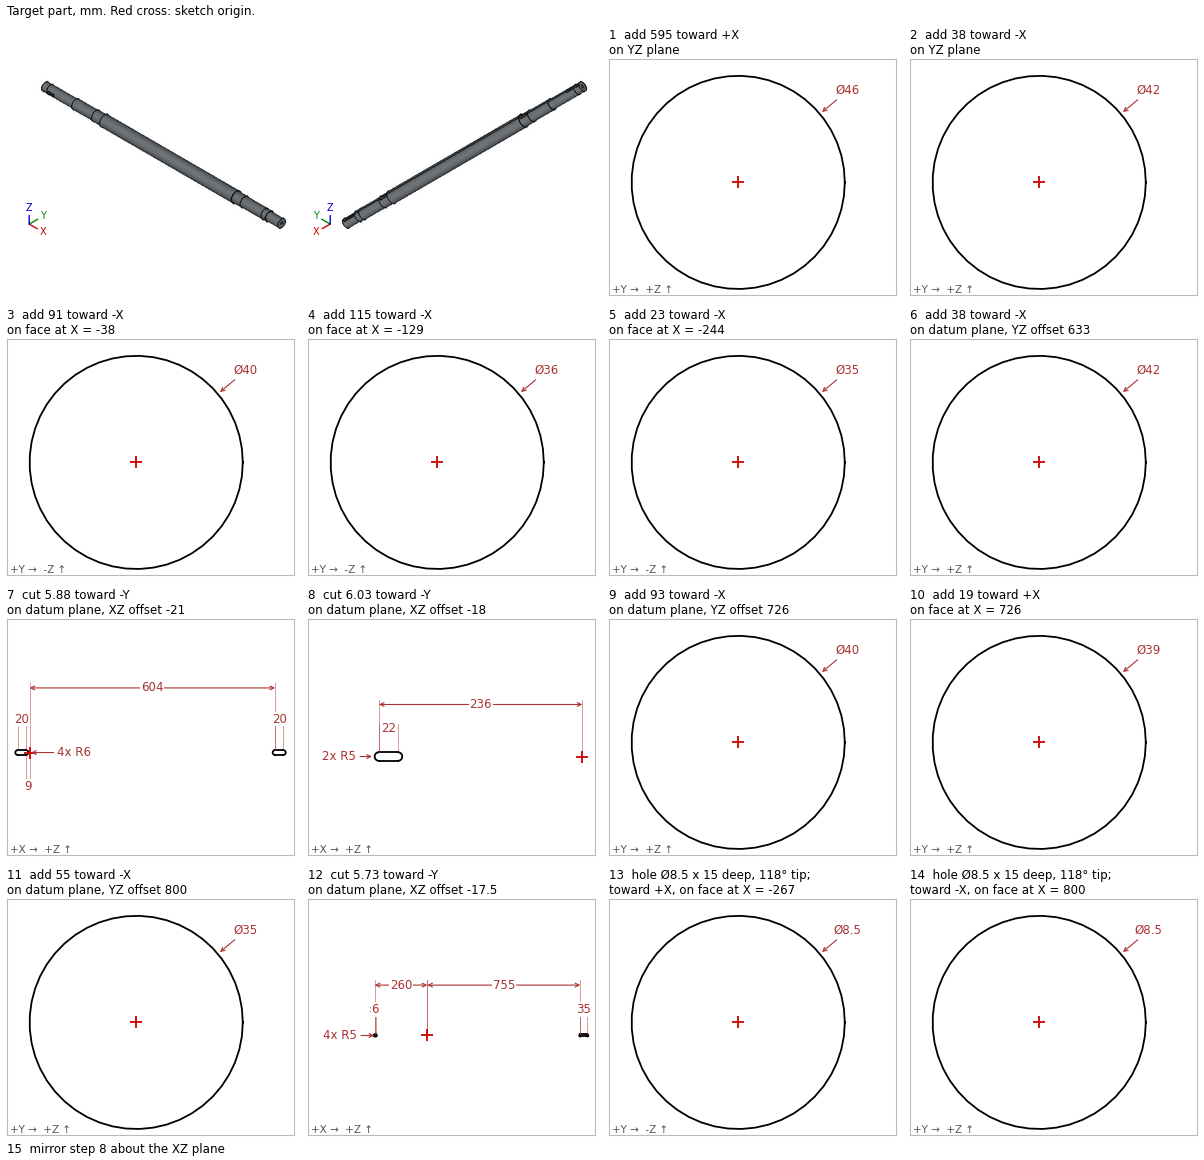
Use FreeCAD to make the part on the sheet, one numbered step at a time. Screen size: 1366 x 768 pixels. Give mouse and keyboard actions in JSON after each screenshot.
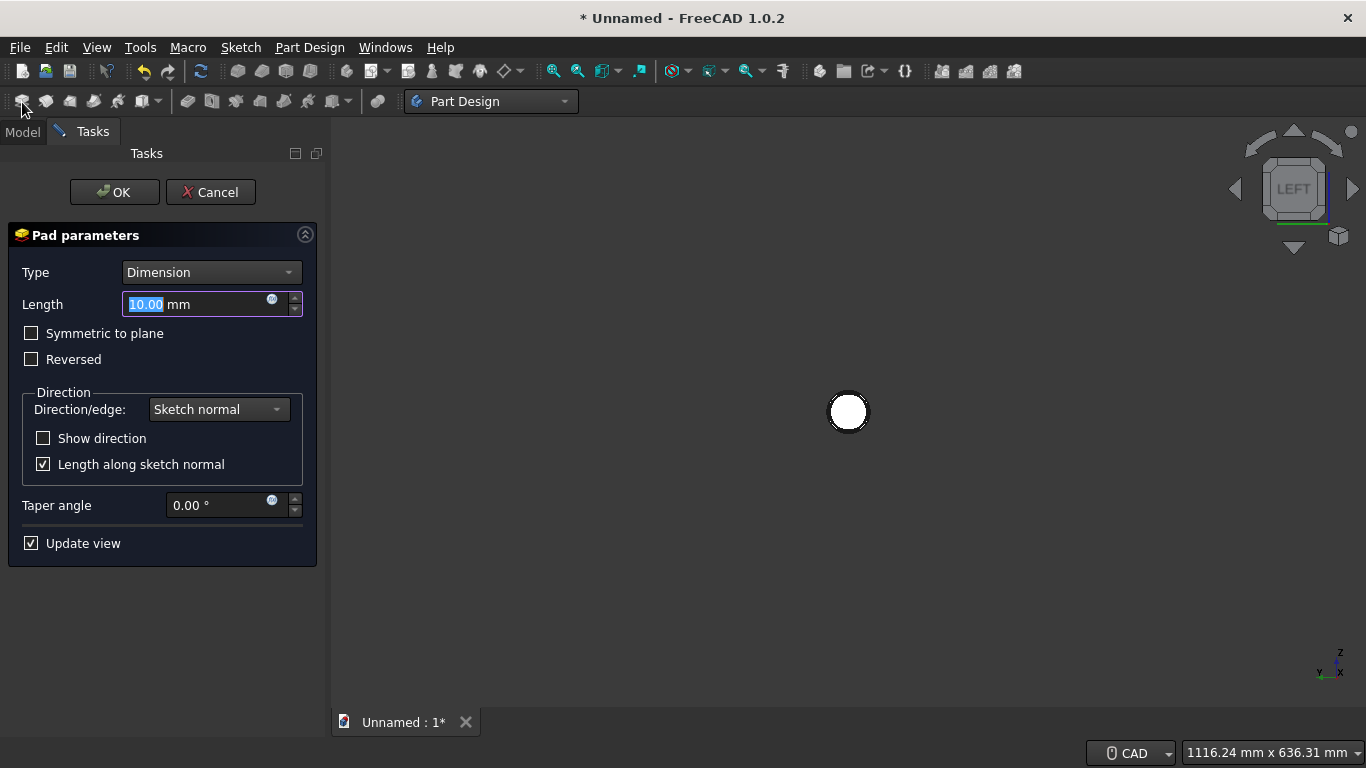
{"action": "type", "text": "91"}
{"action": "key", "text": "Tab"}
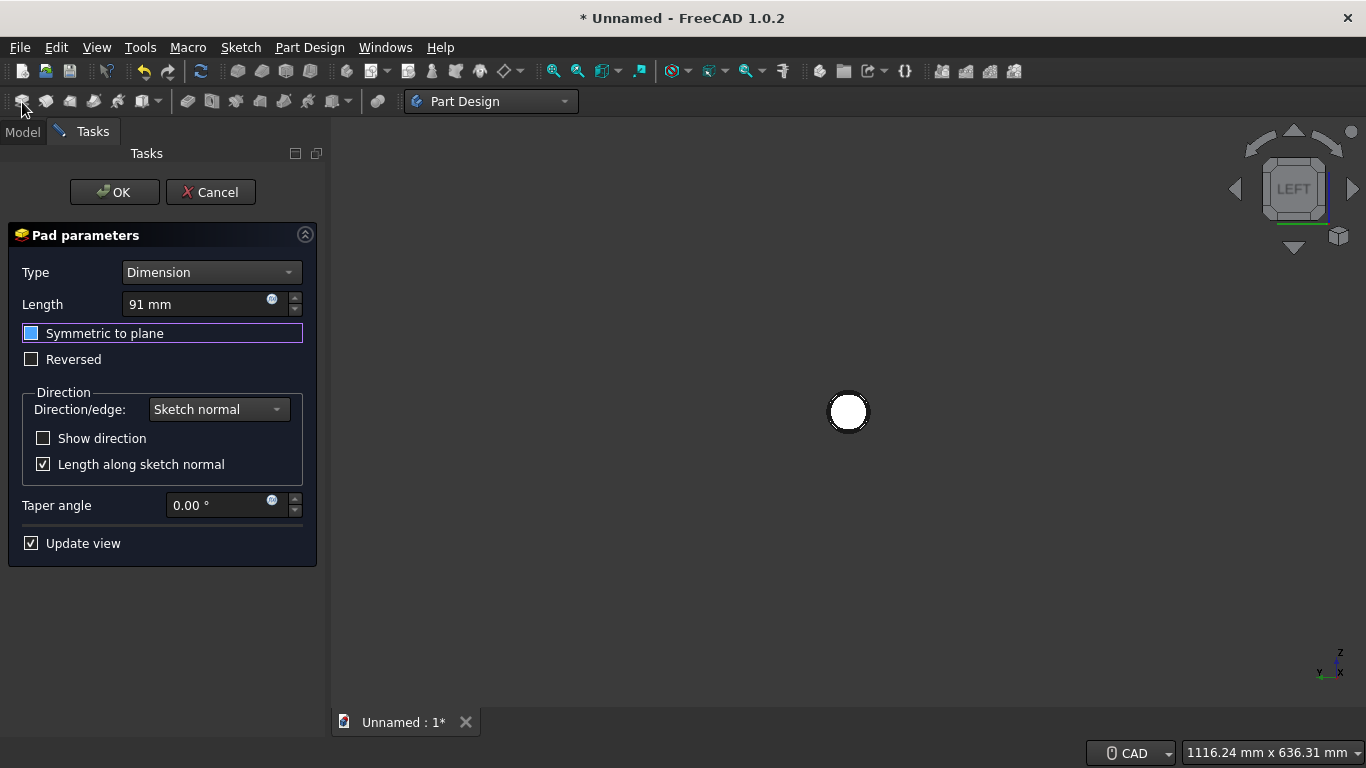
{"action": "left_click", "coordinate": [115, 192]}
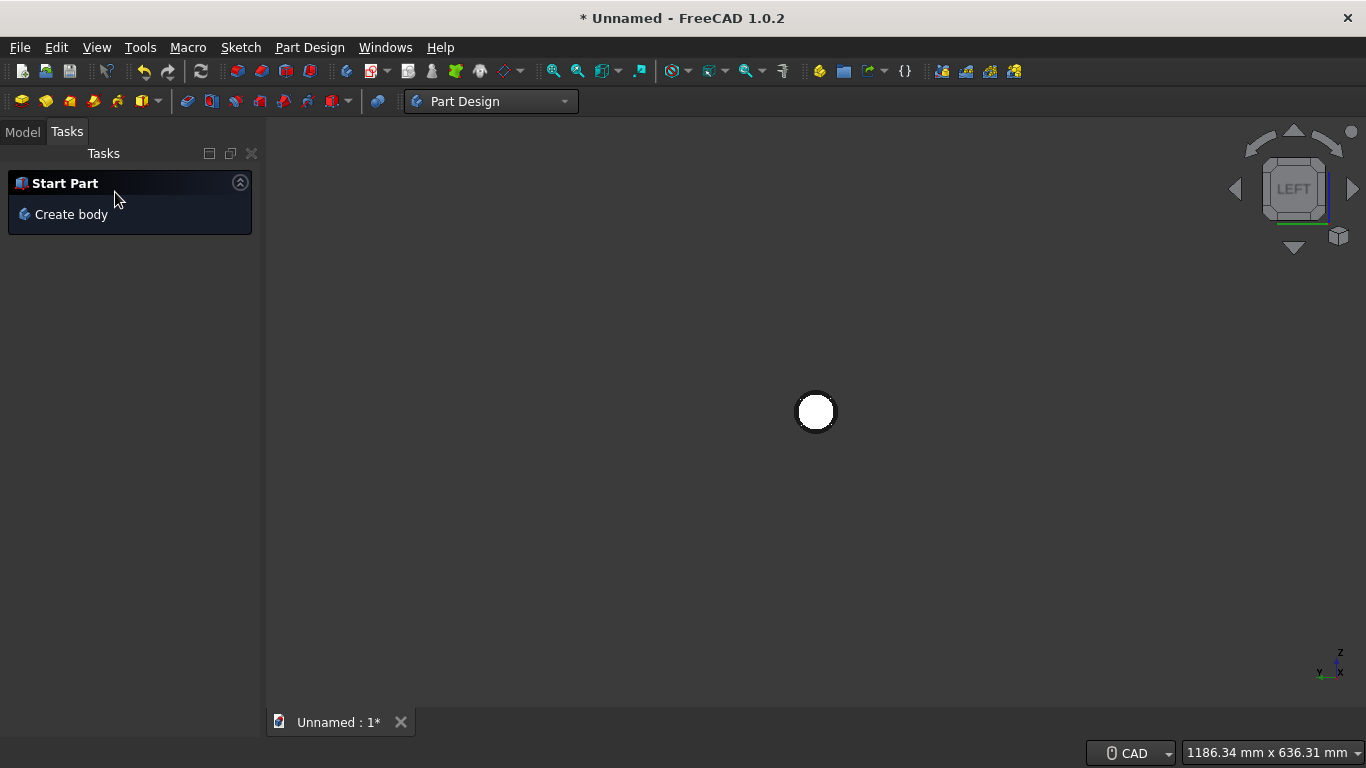
{"action": "key", "text": "v f"}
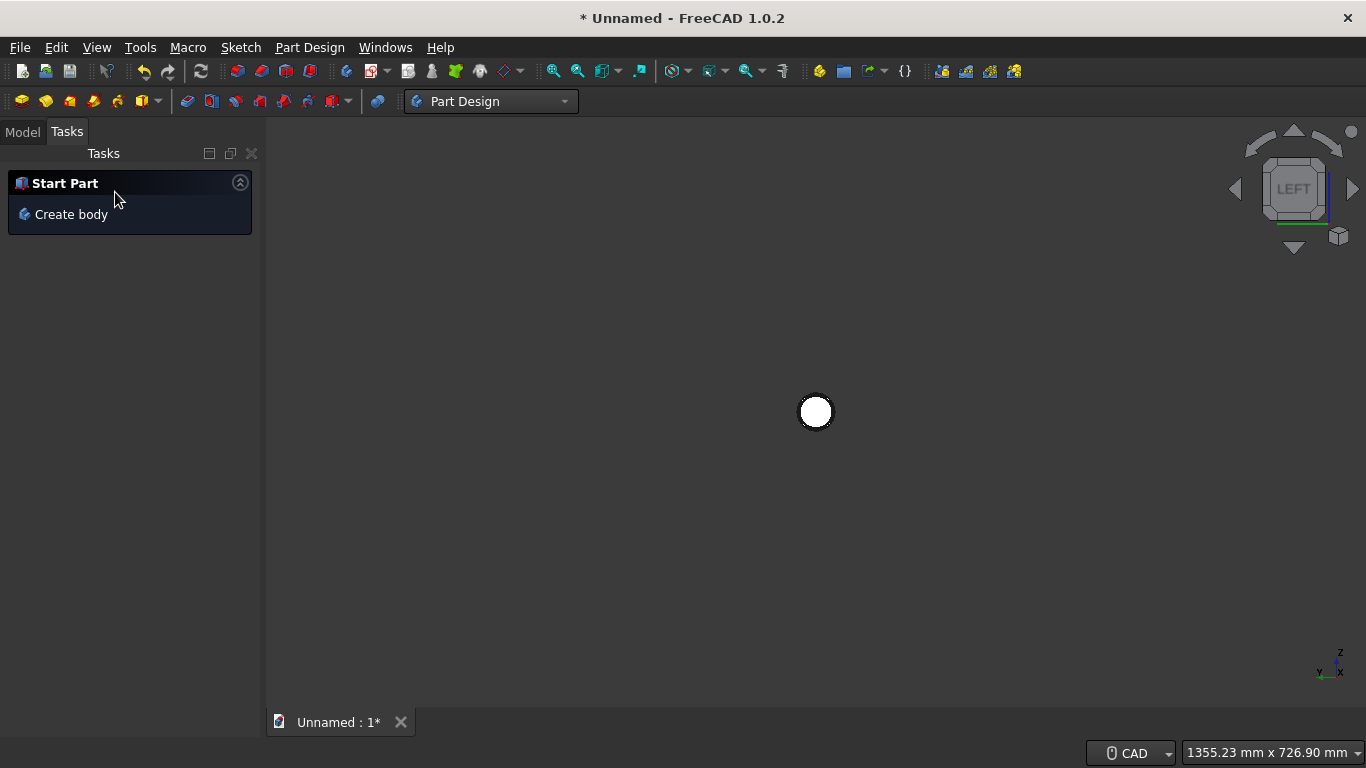
{"action": "left_click", "coordinate": [816, 411]}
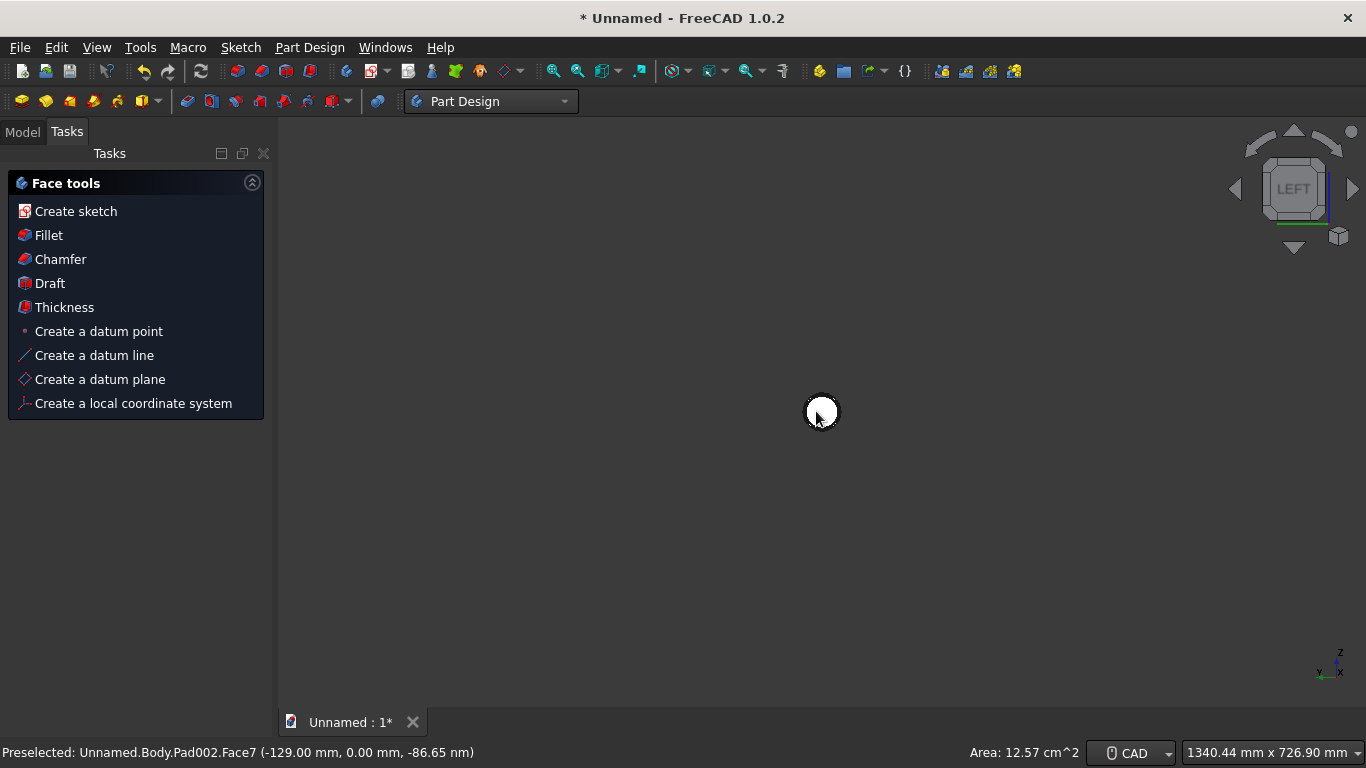
{"action": "left_click", "coordinate": [372, 72]}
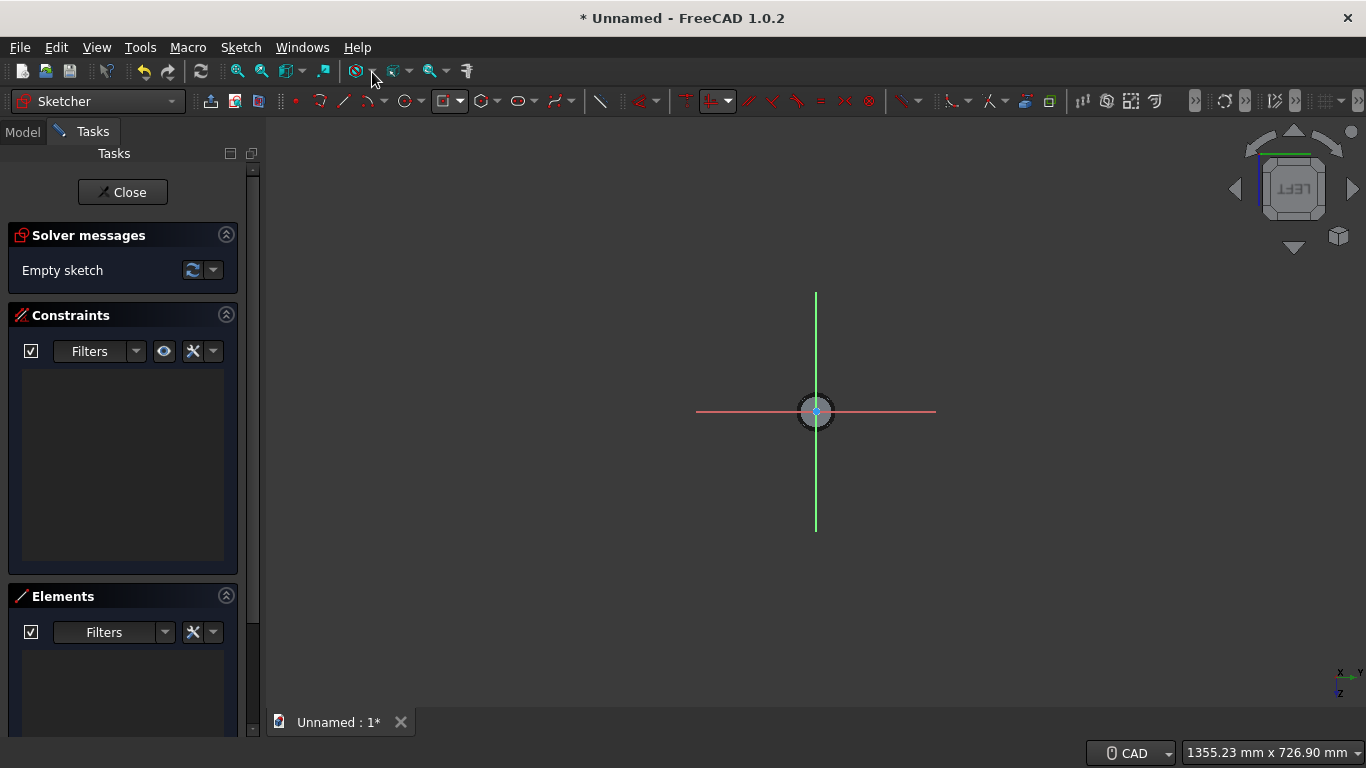
{"action": "scroll", "coordinate": [821, 412], "scroll_direction": "up", "scroll_amount": 13}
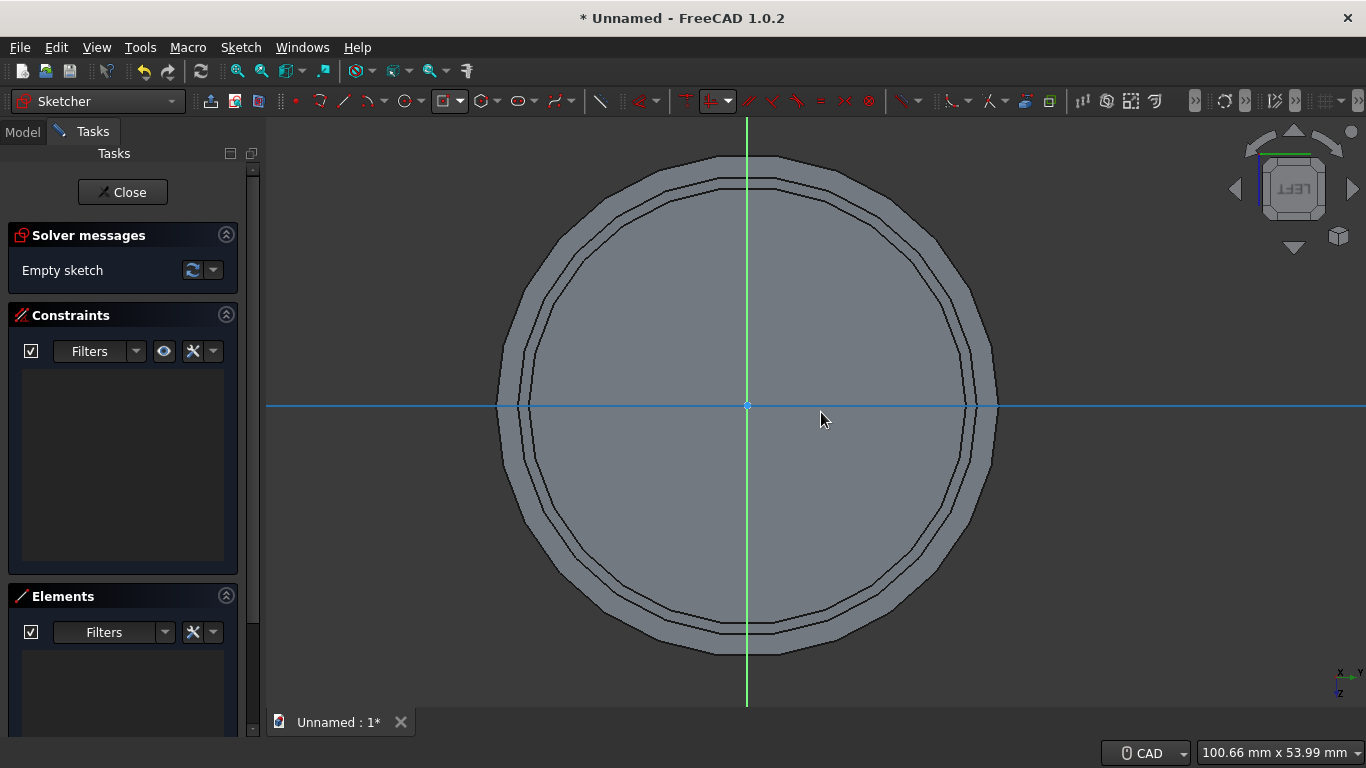
{"action": "key", "text": "g c"}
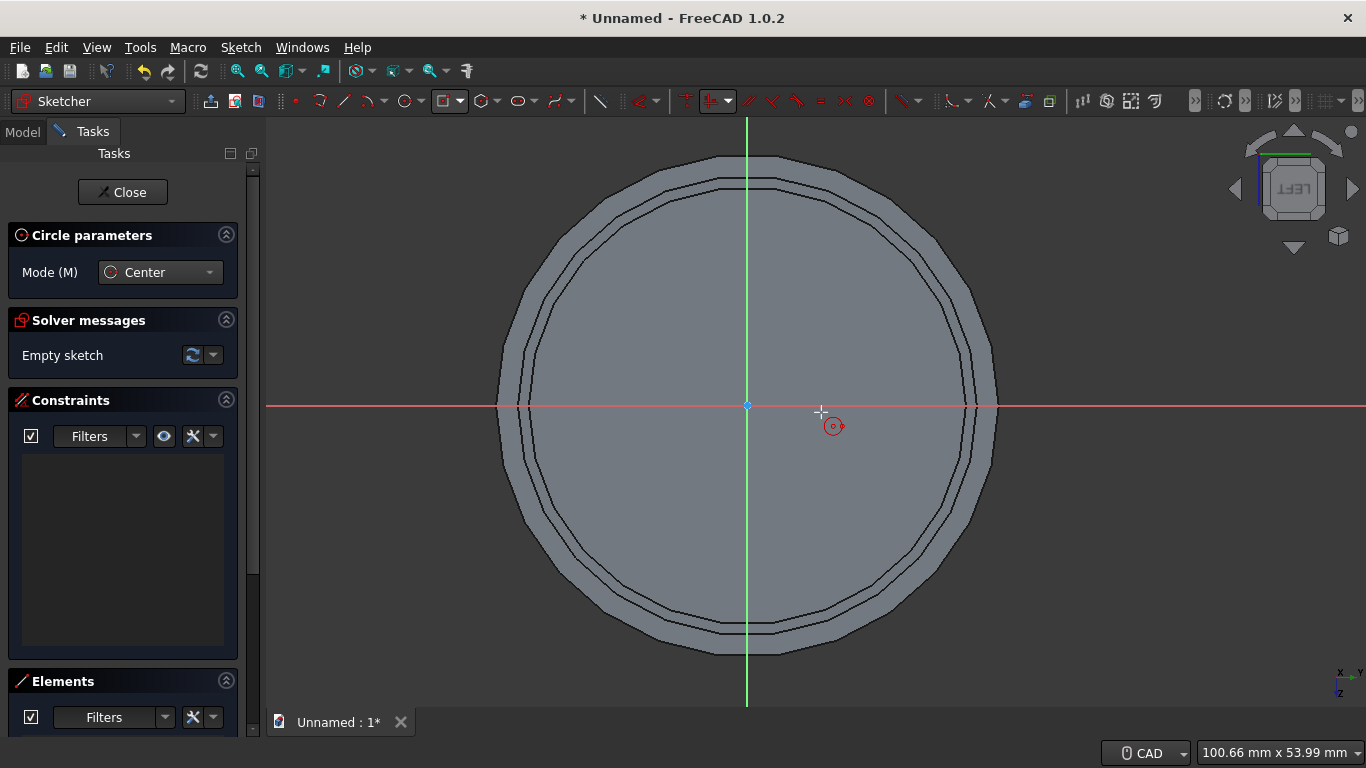
{"action": "left_click", "coordinate": [747, 406]}
{"action": "mouse_move", "coordinate": [886, 267]}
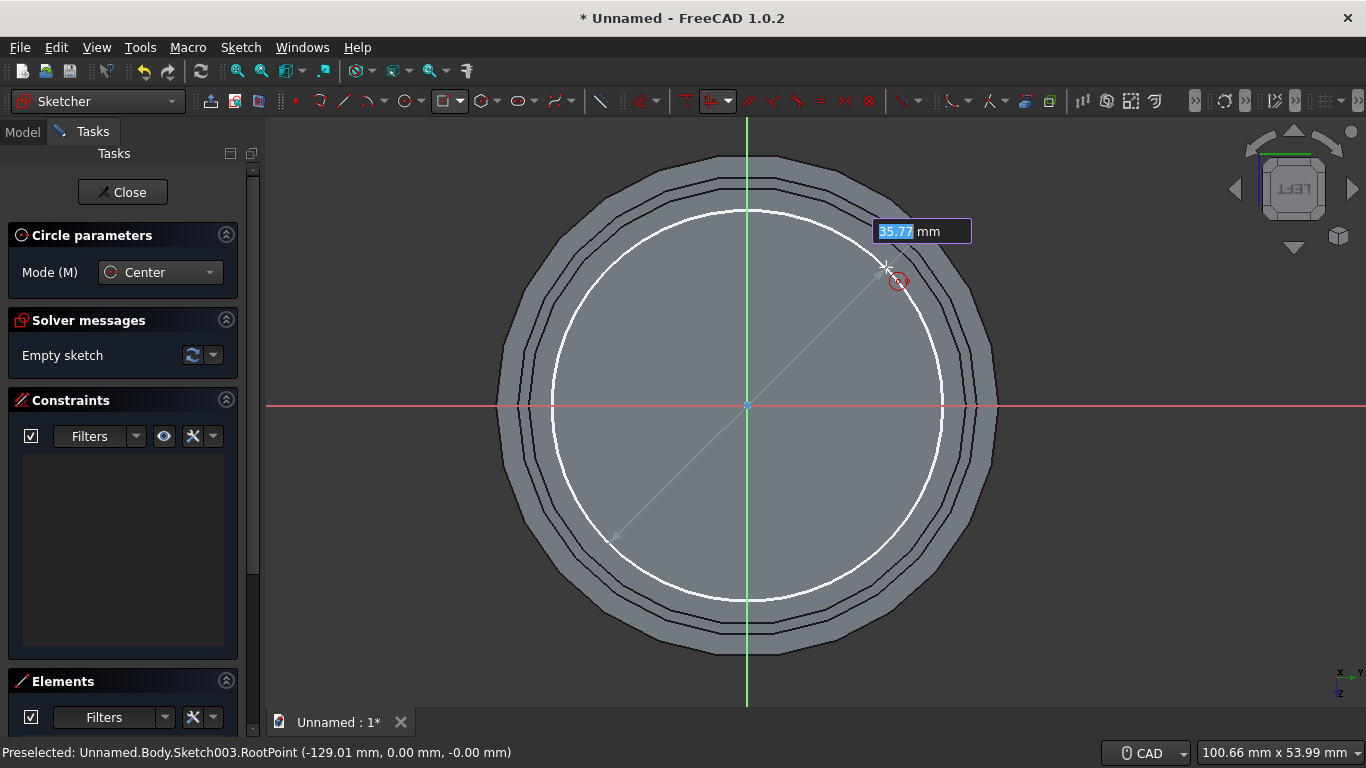
{"action": "type", "text": "36"}
{"action": "key", "text": "Return"}
{"action": "key", "text": "Escape"}